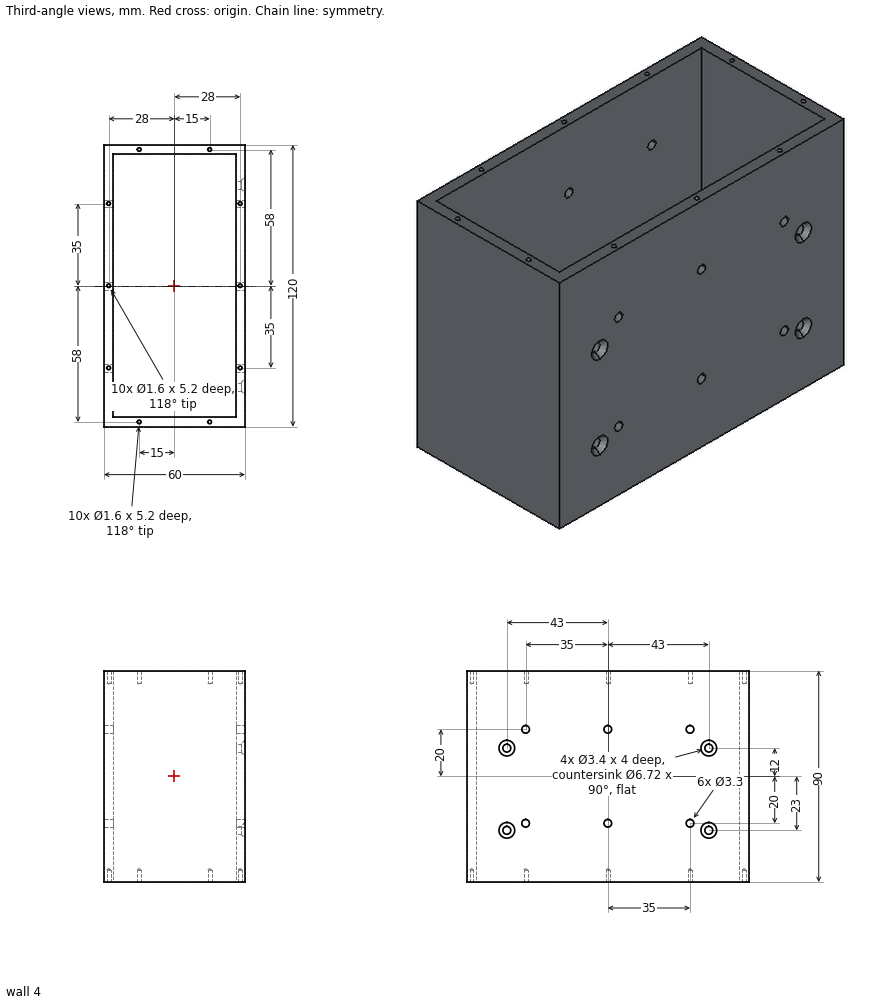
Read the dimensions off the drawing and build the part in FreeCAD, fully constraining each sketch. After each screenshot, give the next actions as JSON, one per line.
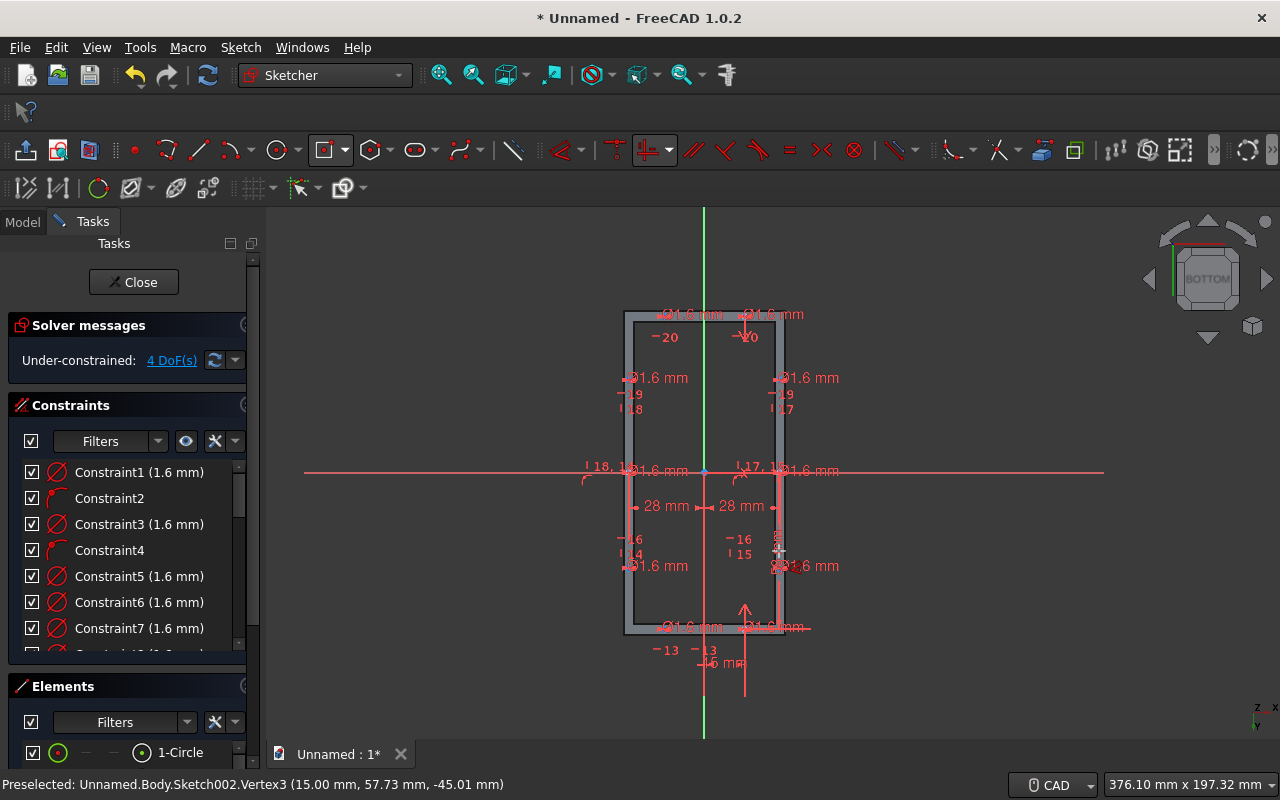
{"action": "left_click", "coordinate": [664, 629]}
{"action": "left_click", "coordinate": [684, 439]}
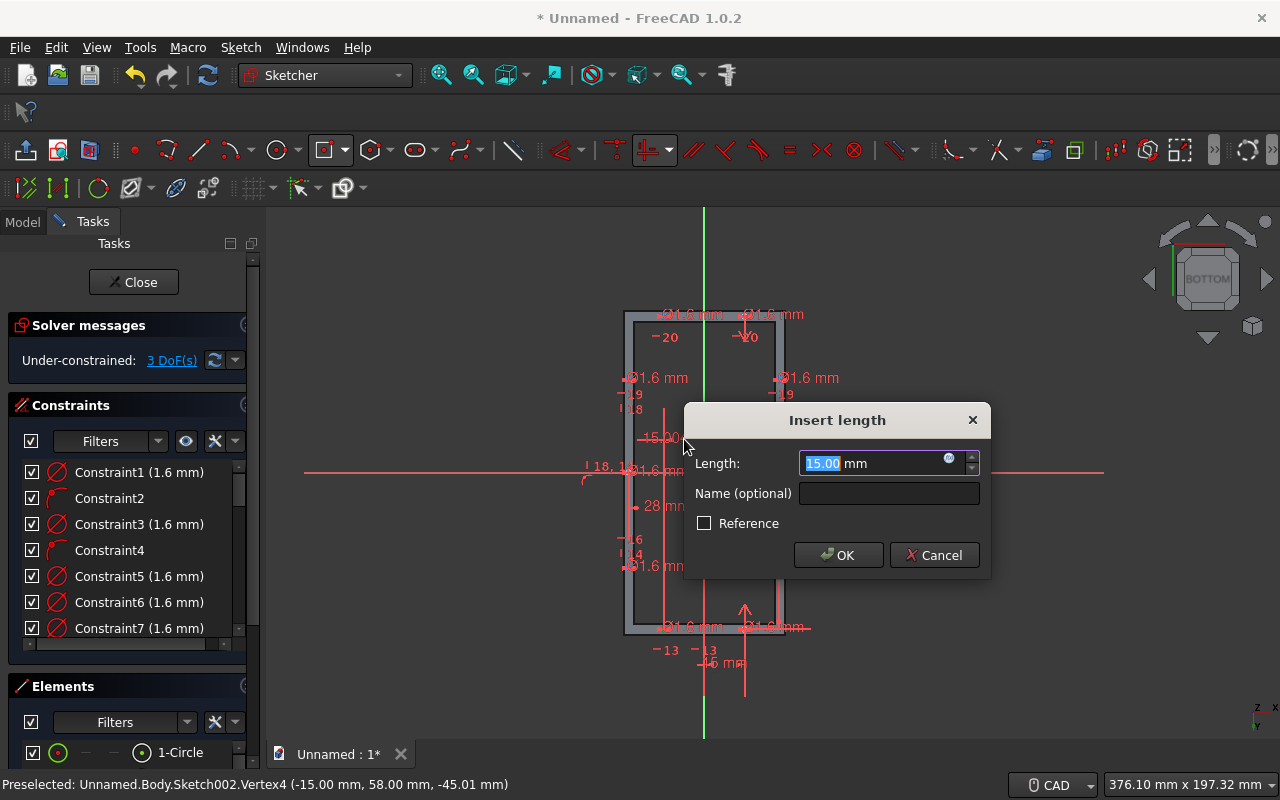
{"action": "type", "text": "15"}
{"action": "key", "text": "Return"}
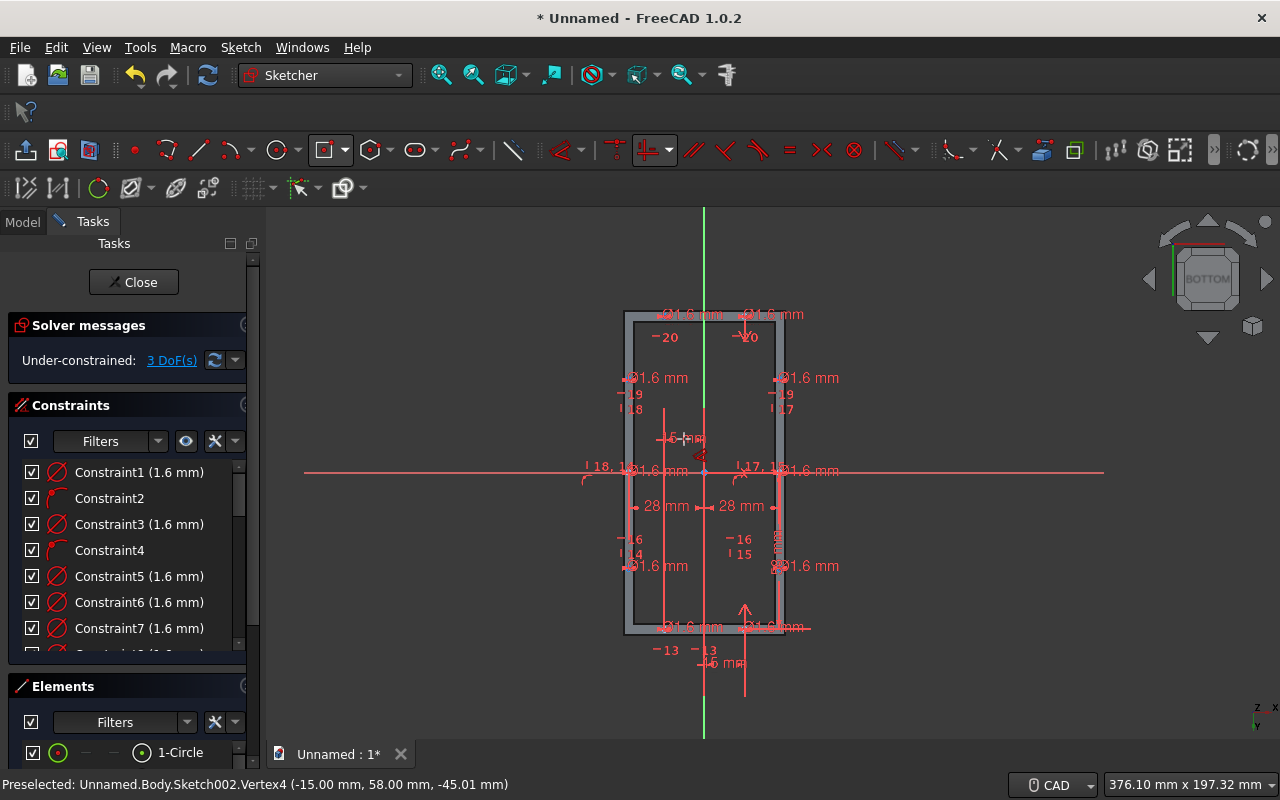
{"action": "left_click", "coordinate": [629, 568]}
{"action": "left_click", "coordinate": [595, 520]}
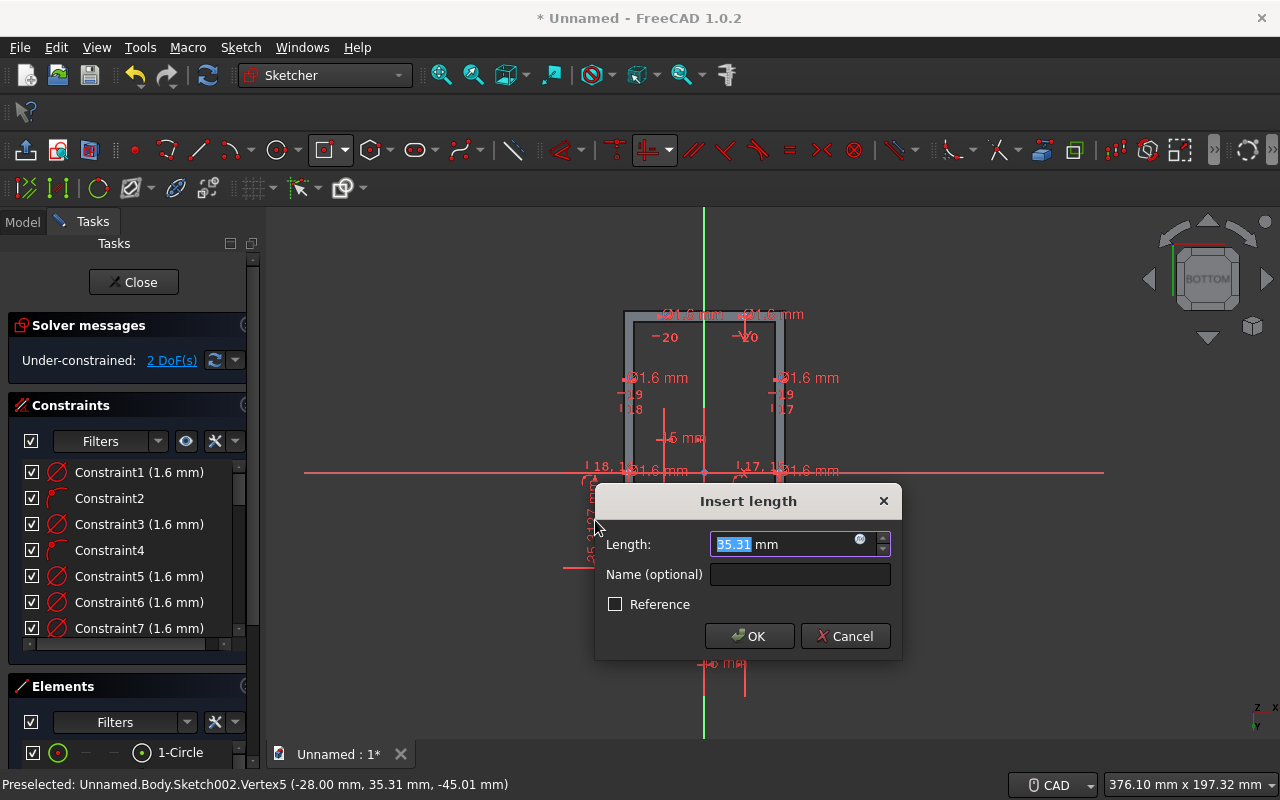
{"action": "type", "text": "35"}
{"action": "key", "text": "Return"}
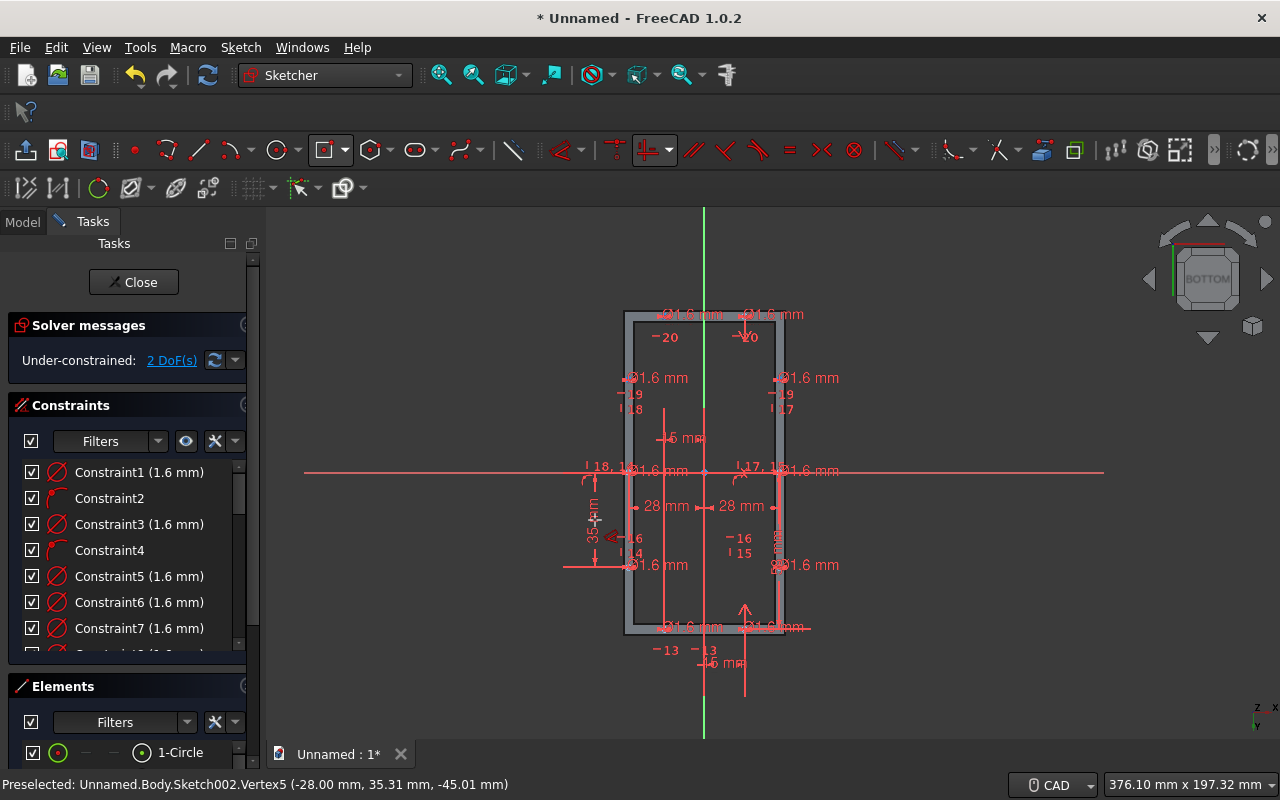
{"action": "left_click", "coordinate": [780, 380]}
{"action": "left_click", "coordinate": [814, 426]}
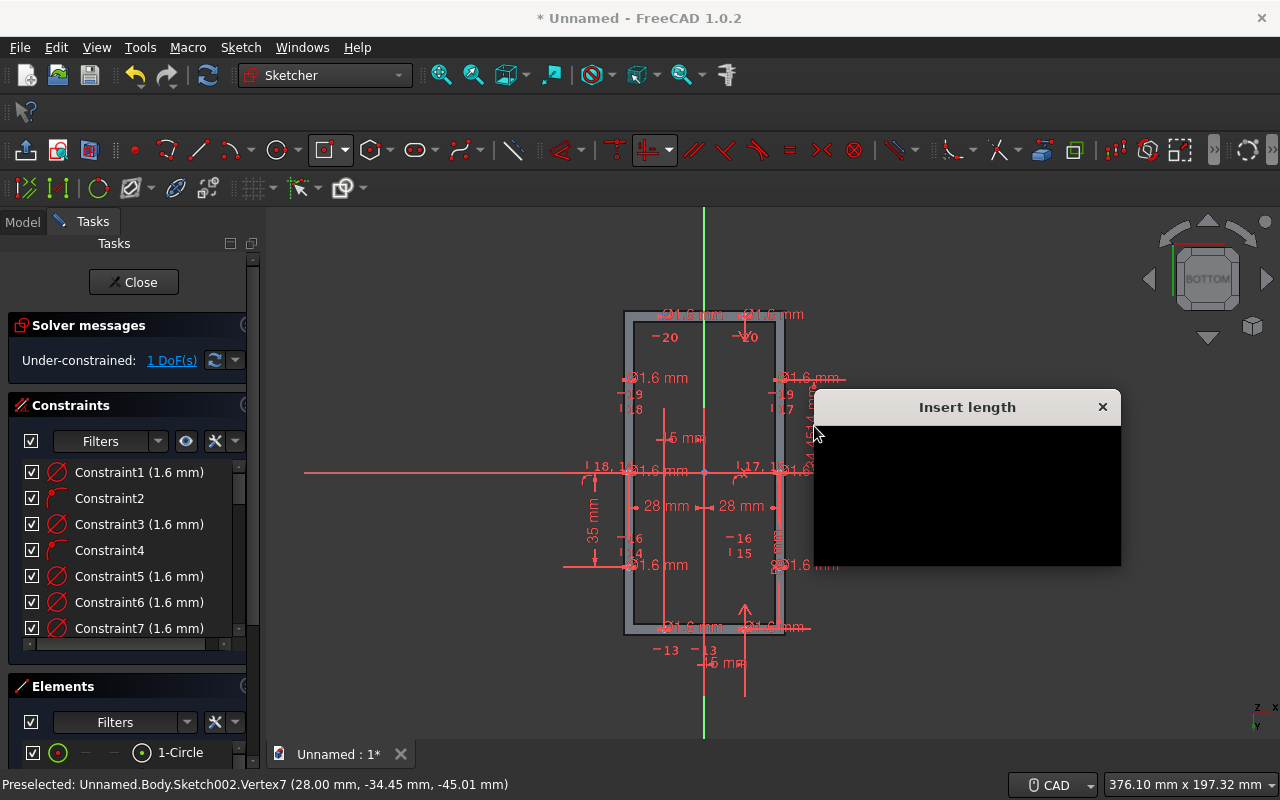
{"action": "type", "text": "35"}
{"action": "key", "text": "Return"}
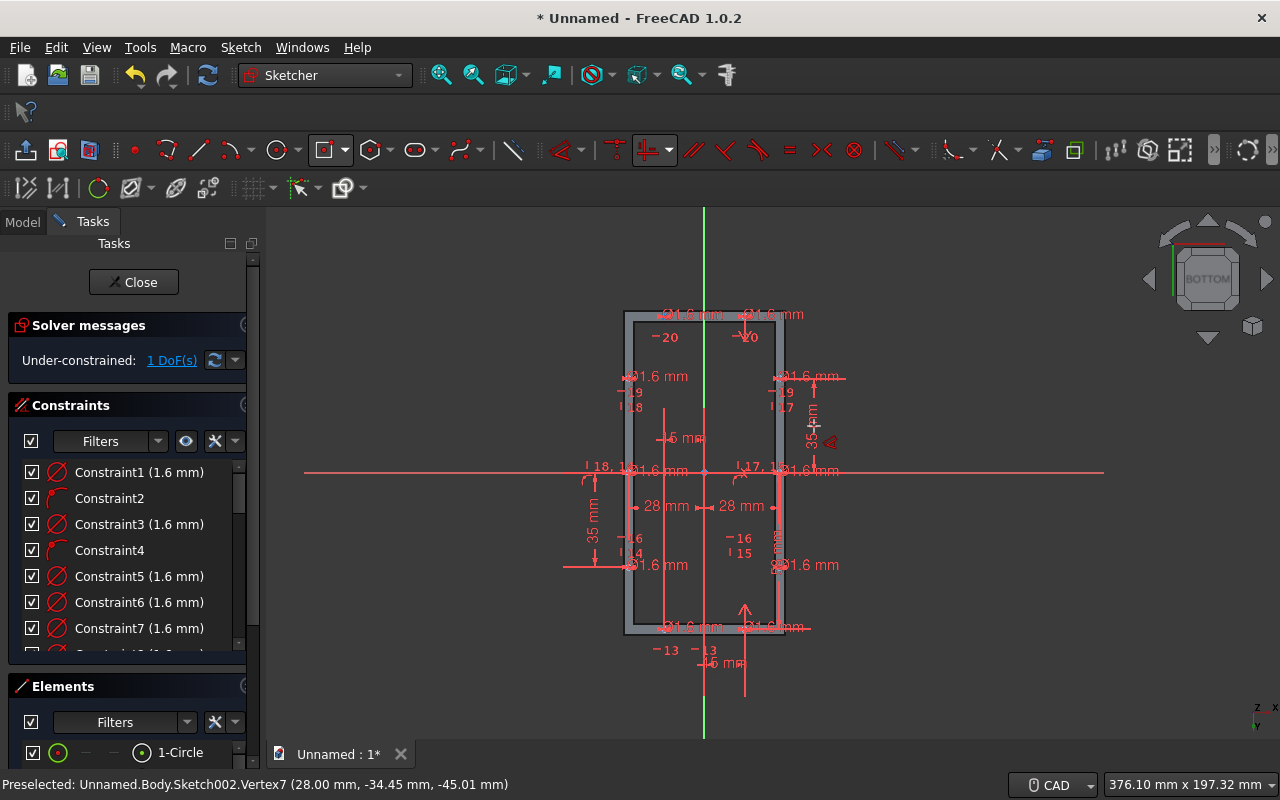
{"action": "left_click", "coordinate": [664, 317]}
{"action": "left_click", "coordinate": [684, 283]}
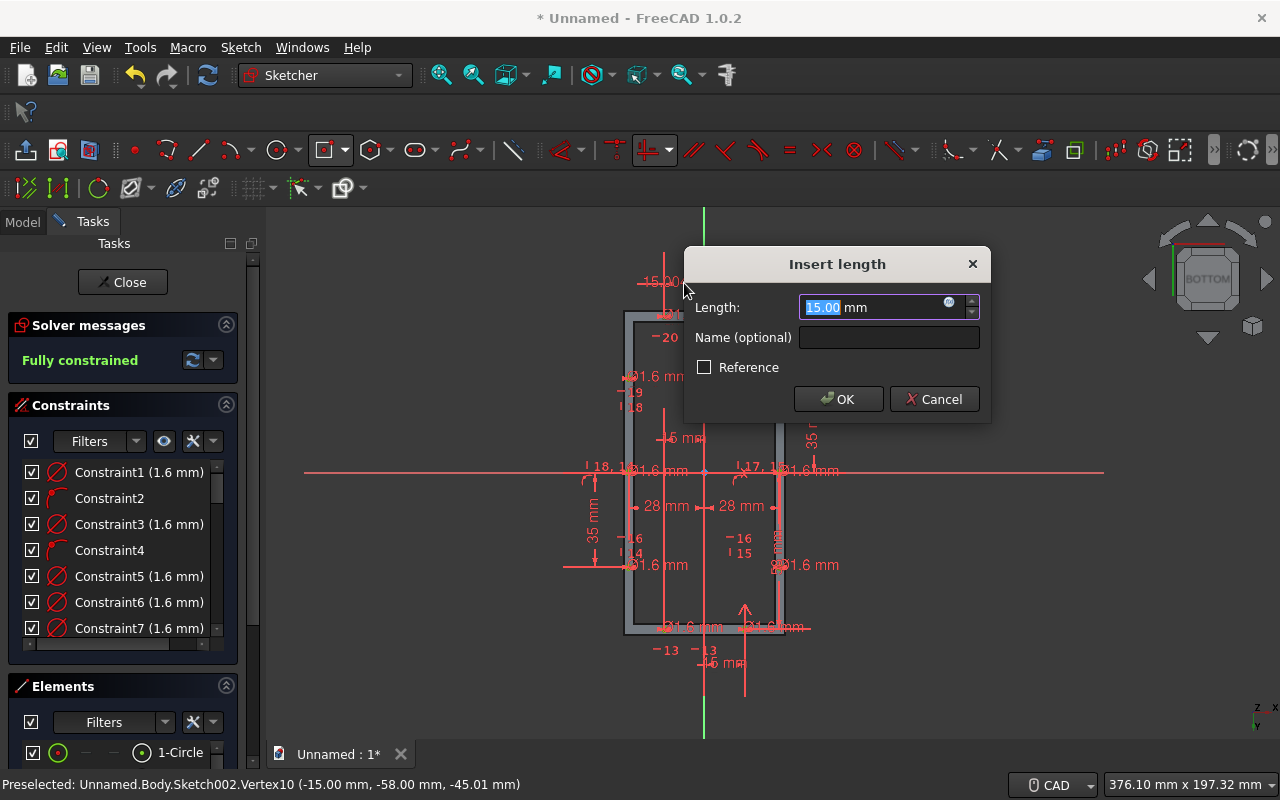
{"action": "type", "text": "15"}
{"action": "key", "text": "Return"}
{"action": "key", "text": "Escape"}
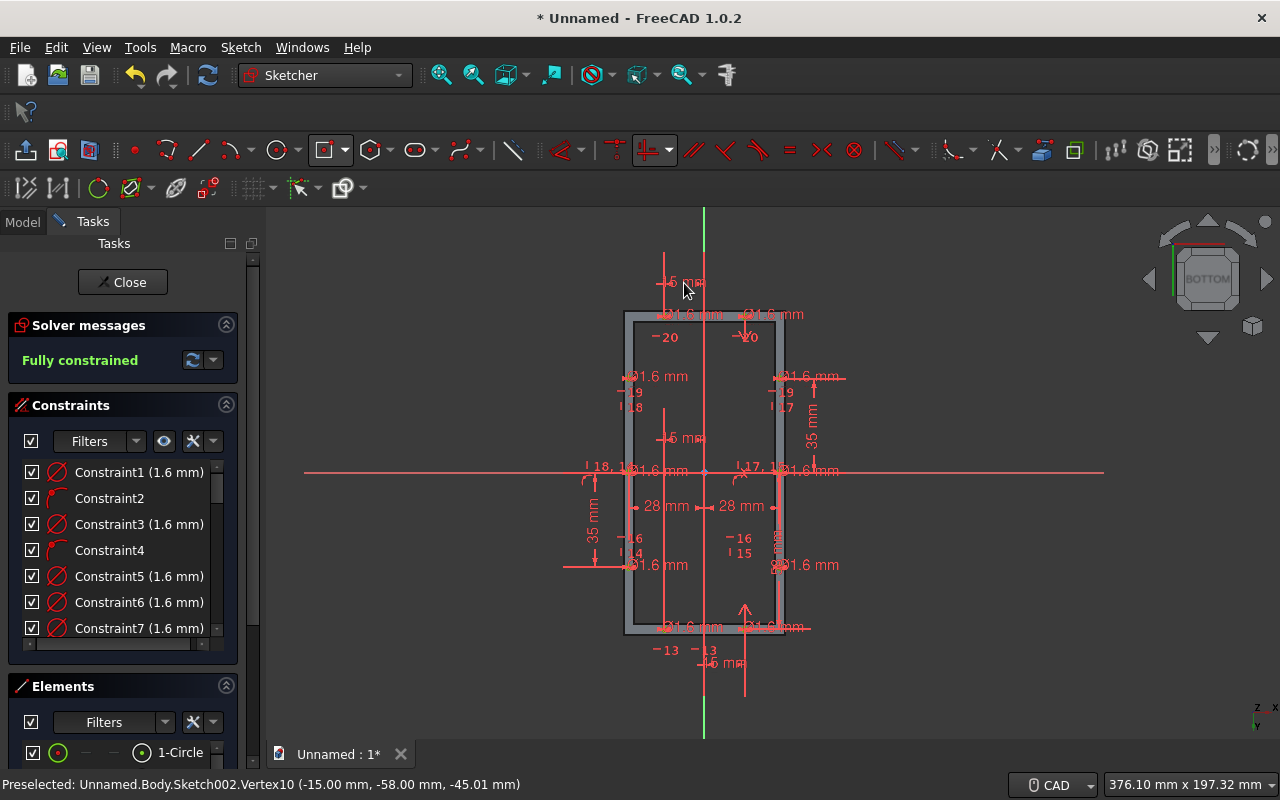
{"action": "left_click", "coordinate": [123, 282]}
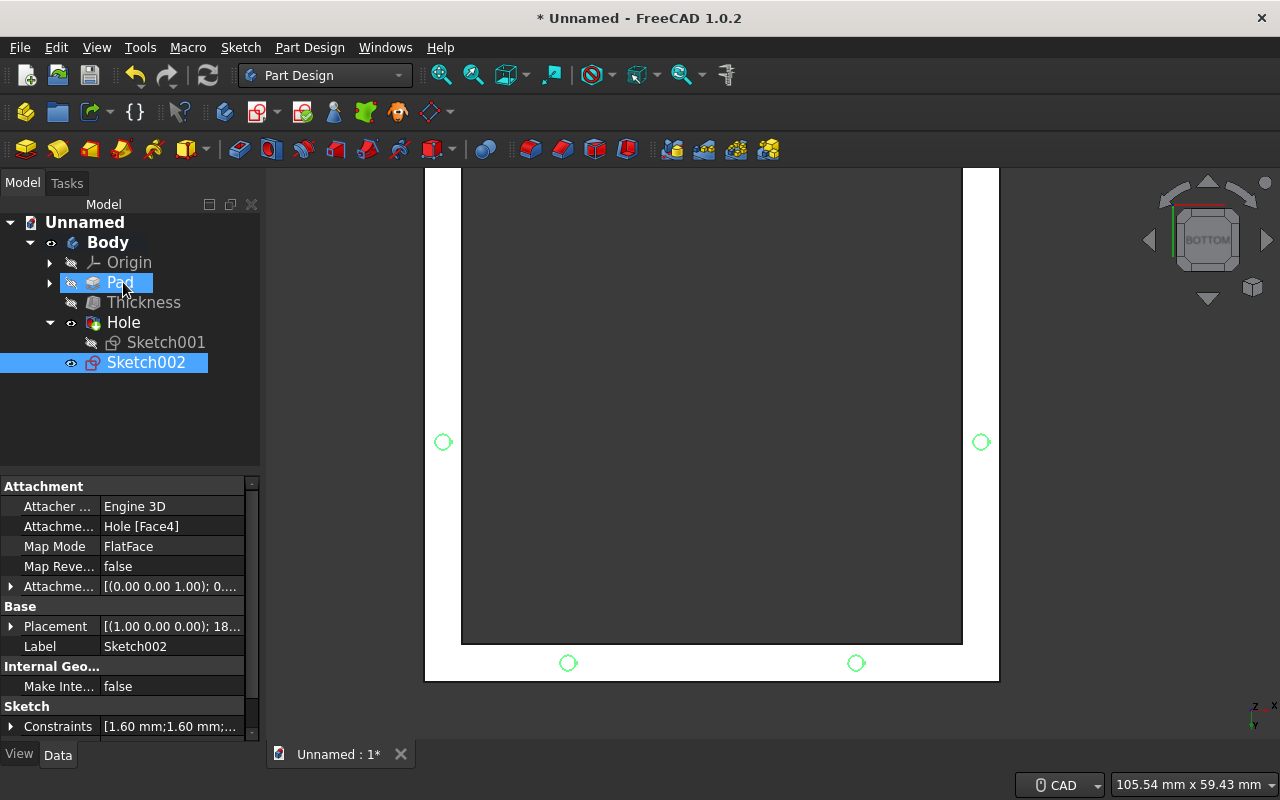
{"action": "left_click", "coordinate": [272, 150]}